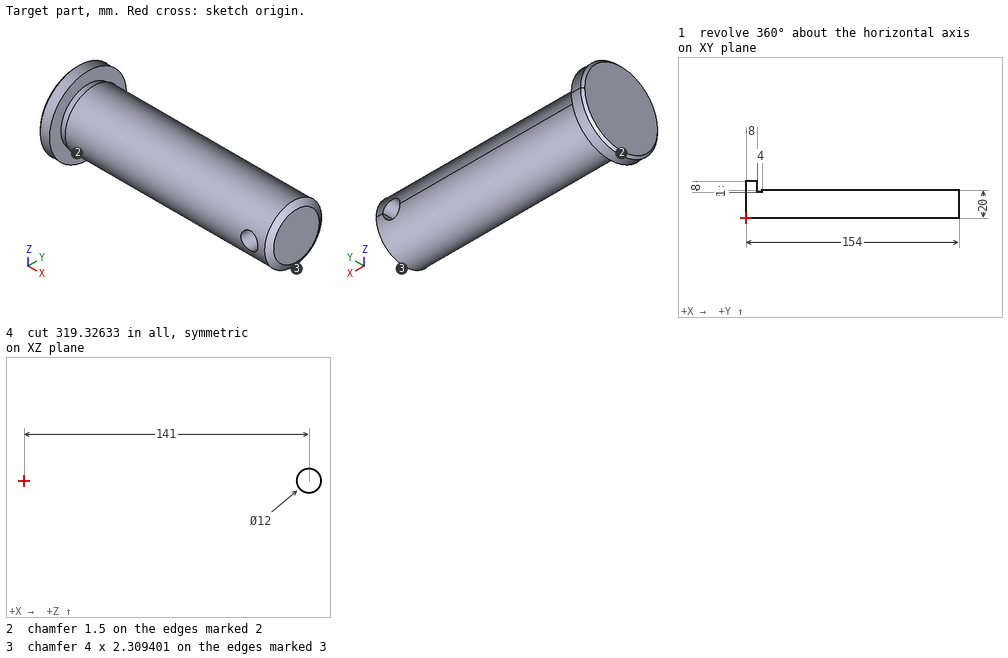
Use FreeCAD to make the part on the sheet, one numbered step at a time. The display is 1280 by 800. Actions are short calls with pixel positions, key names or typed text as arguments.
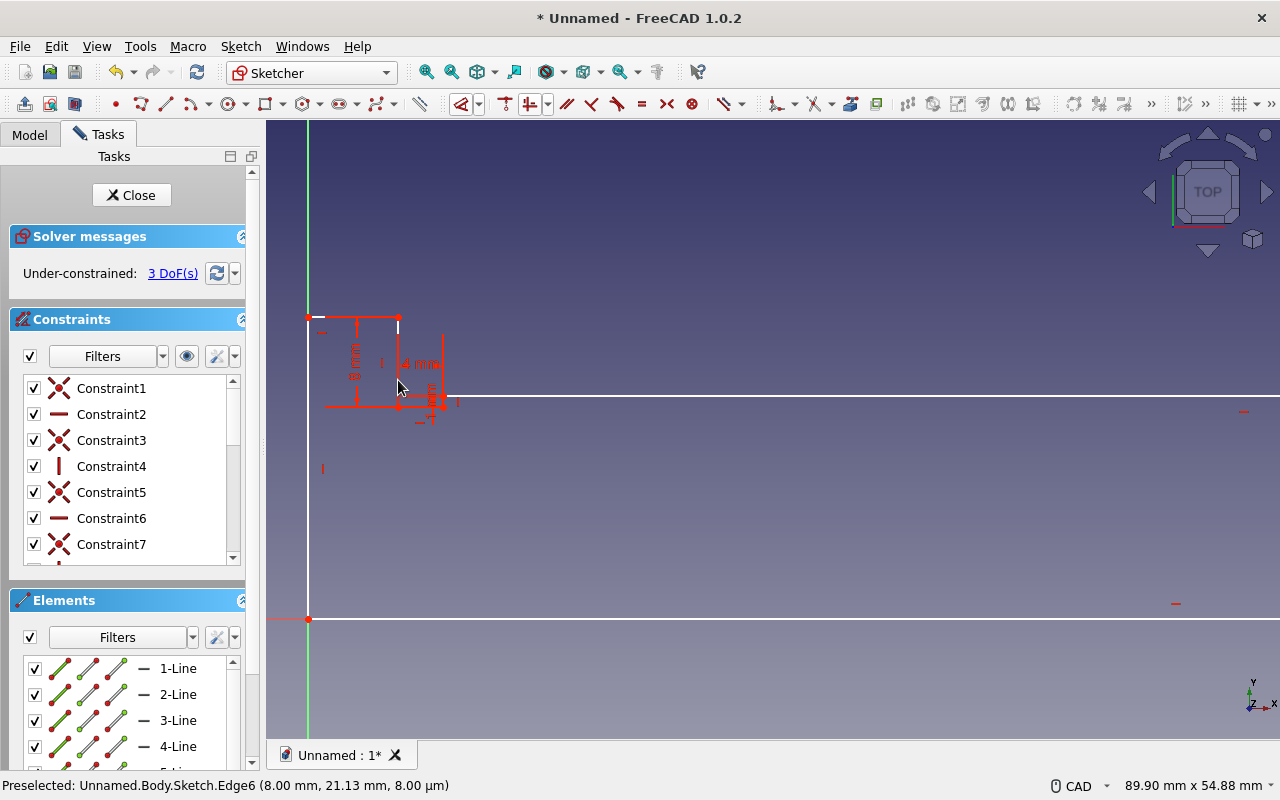
click(371, 317)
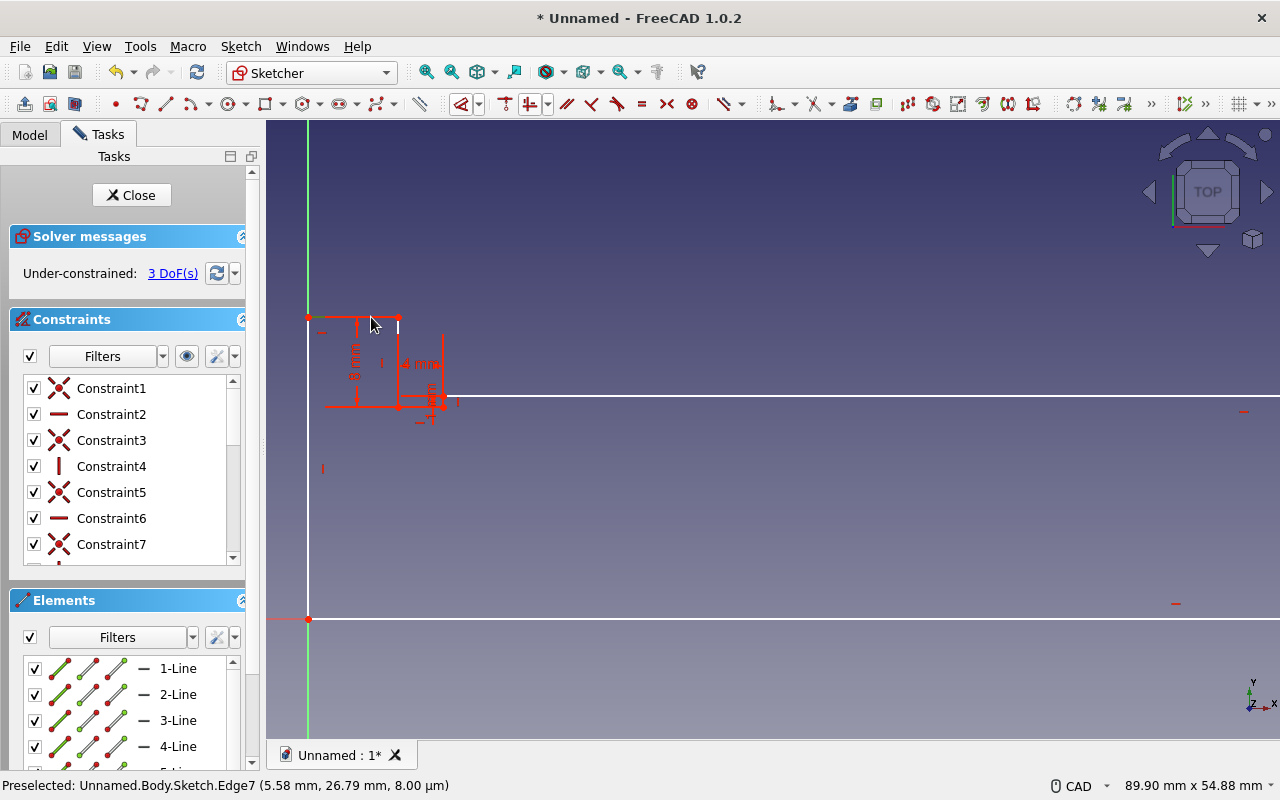
click(478, 104)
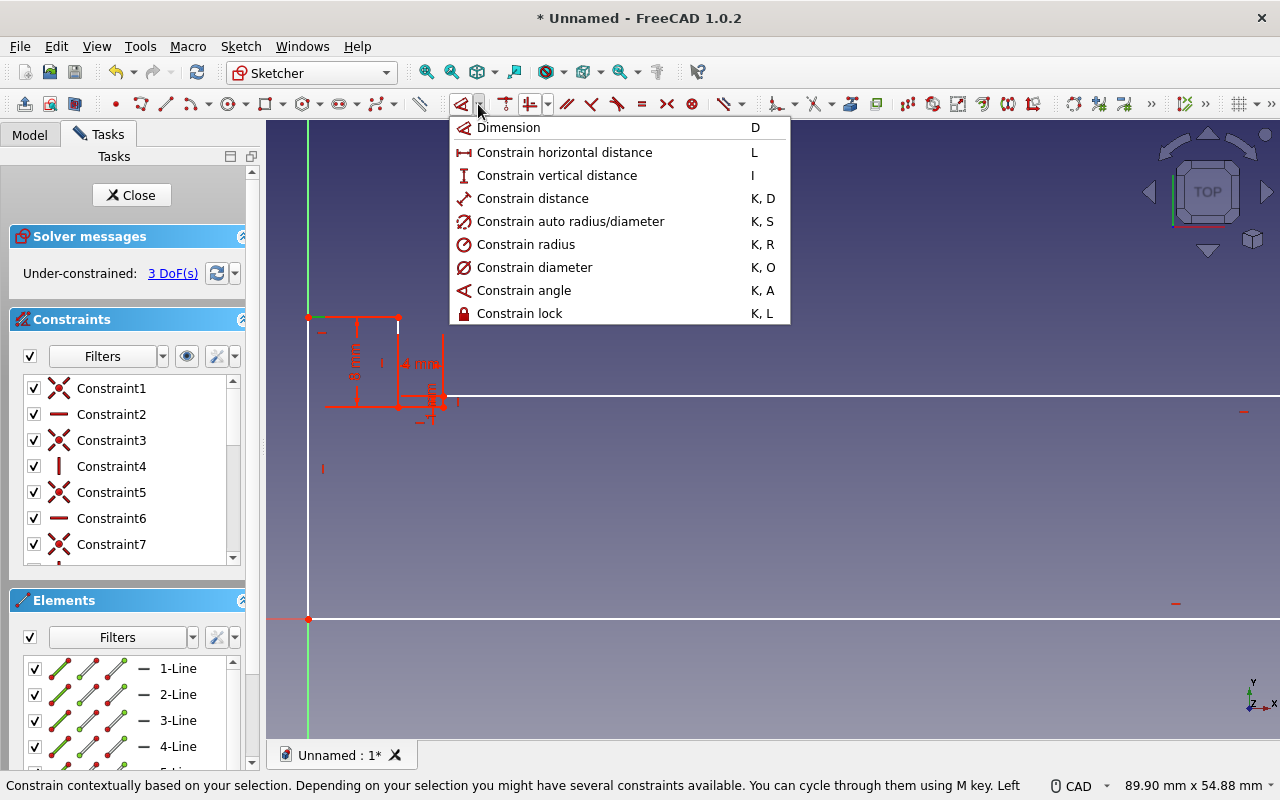
click(620, 152)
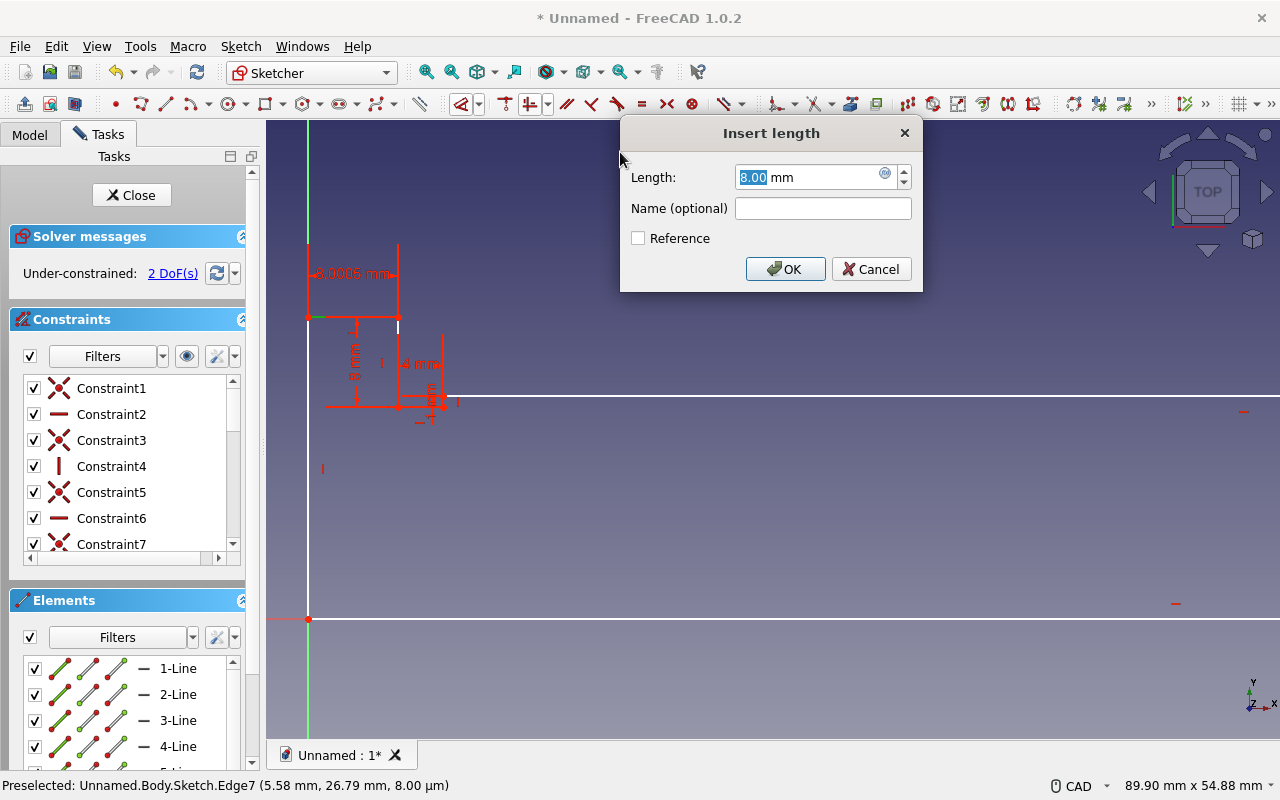
text(8)
key(Return)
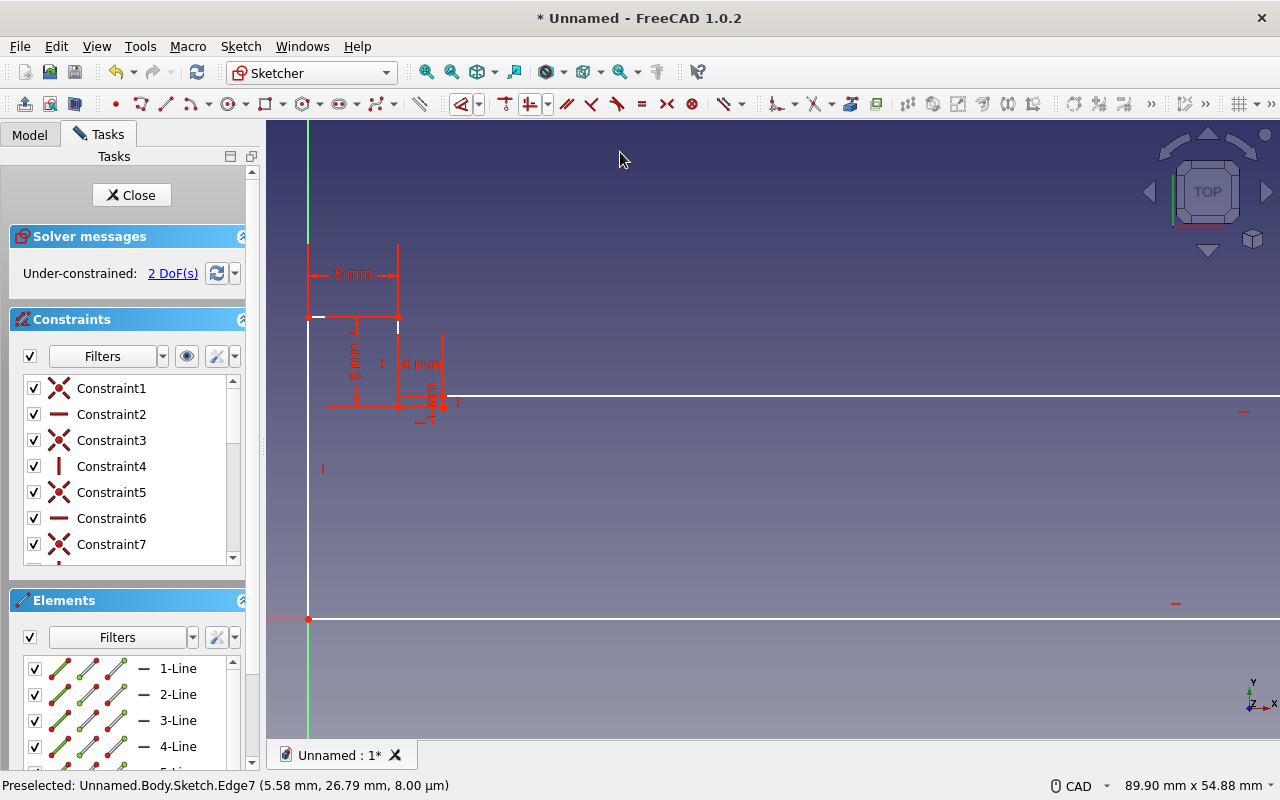
scroll(430, 408, down, 5)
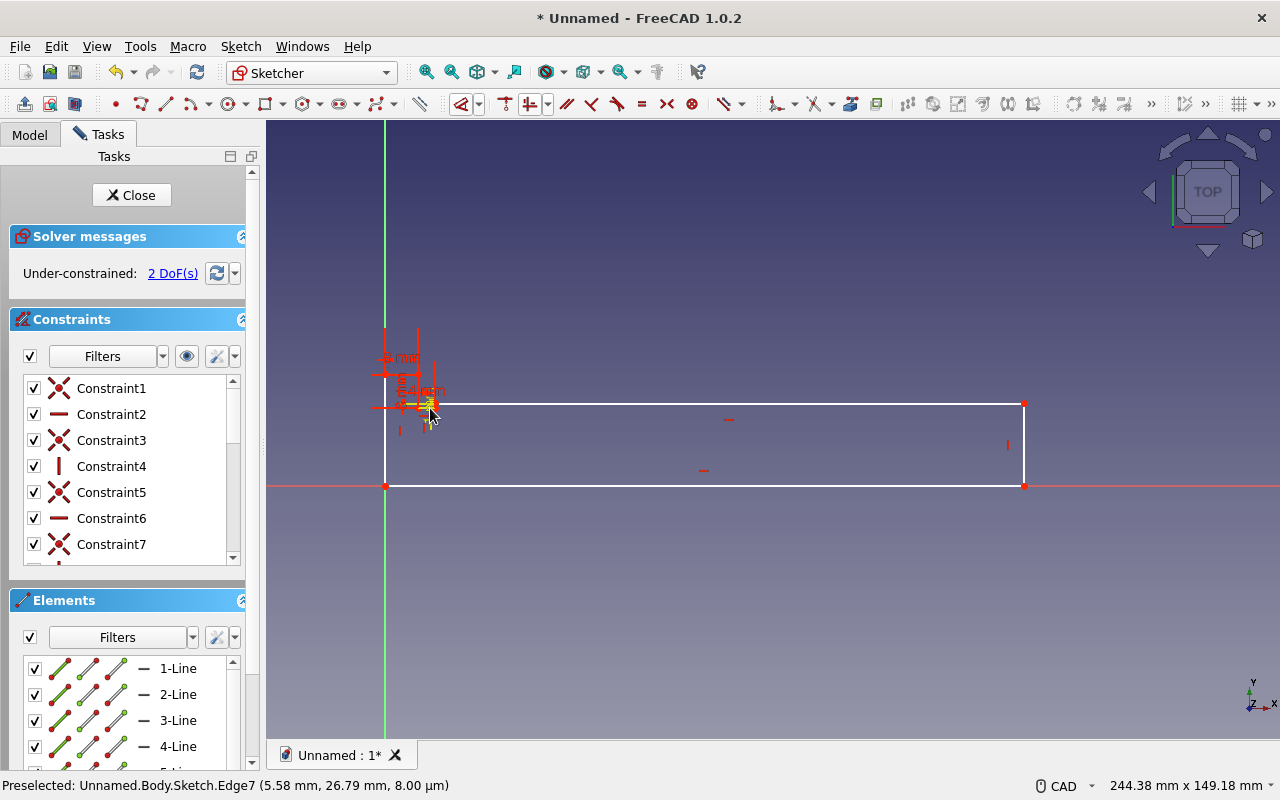
click(1024, 461)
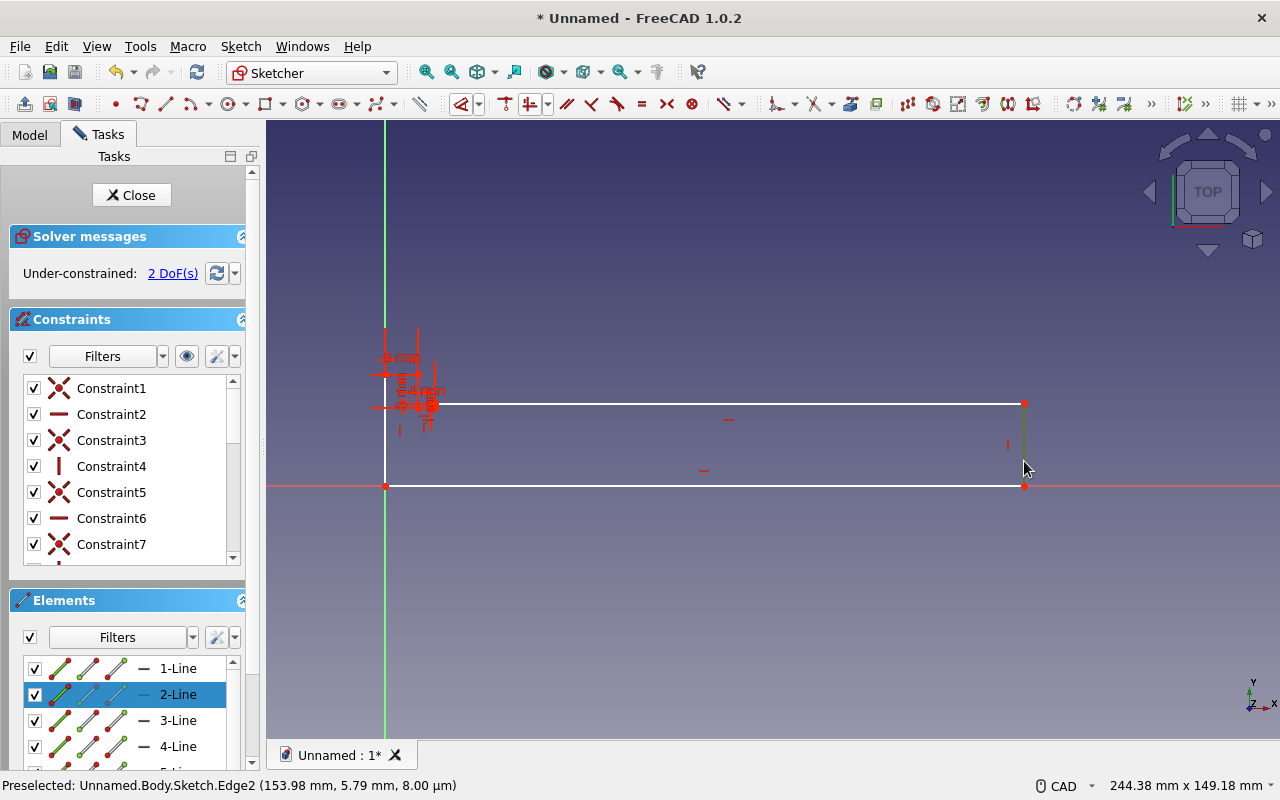
click(478, 104)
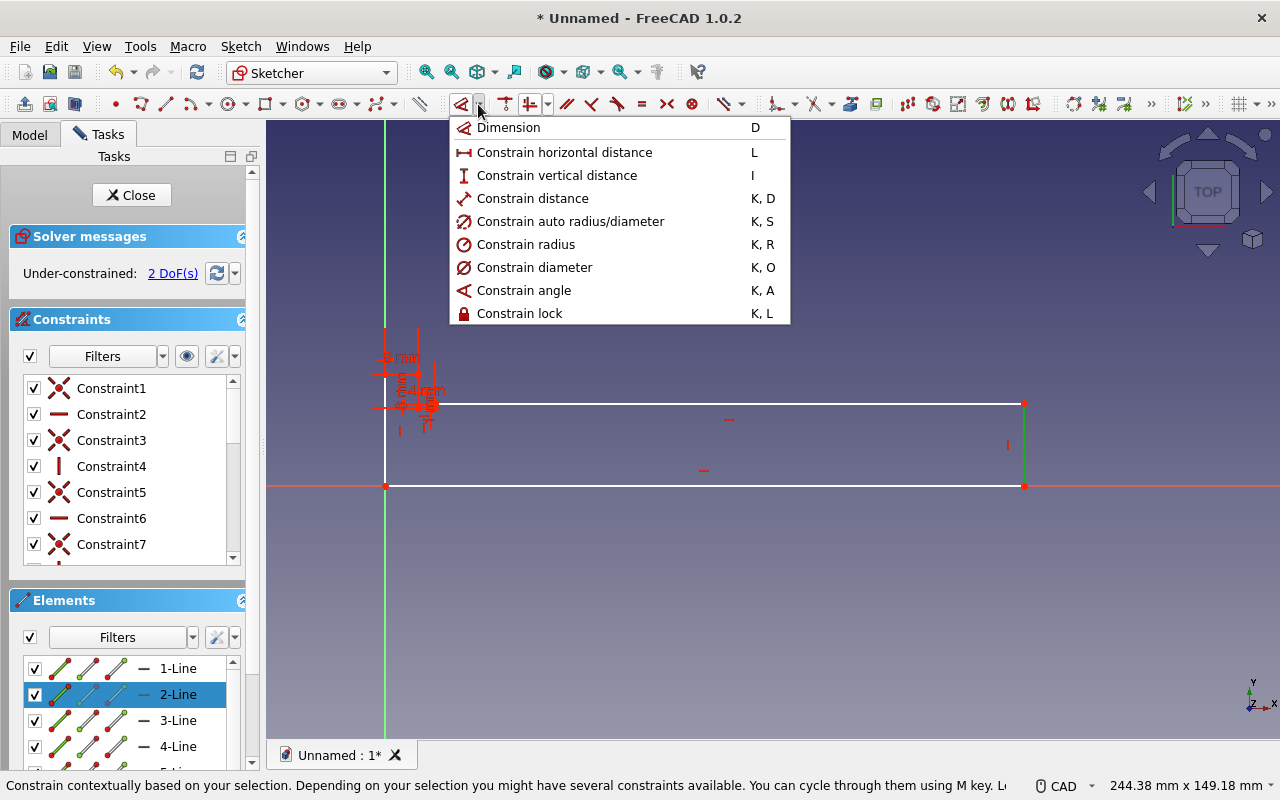
click(620, 176)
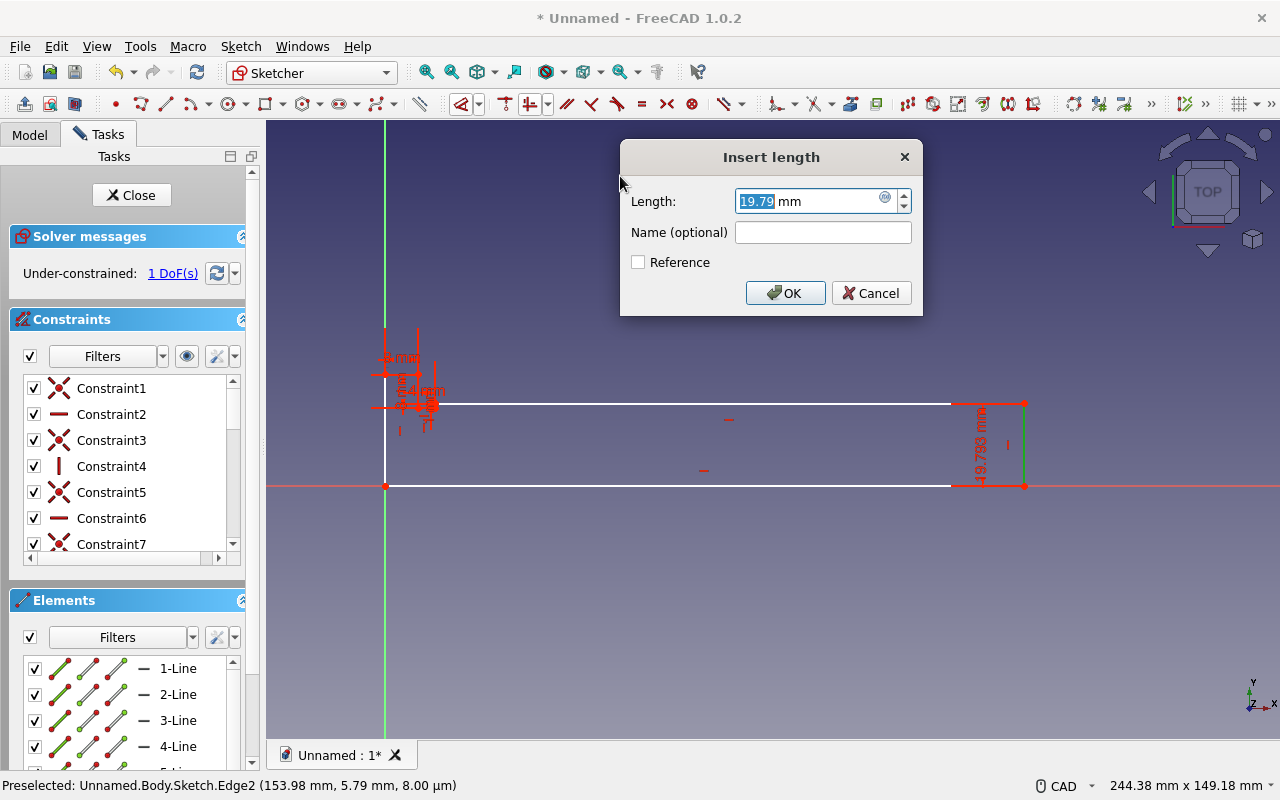
text(20)
key(Return)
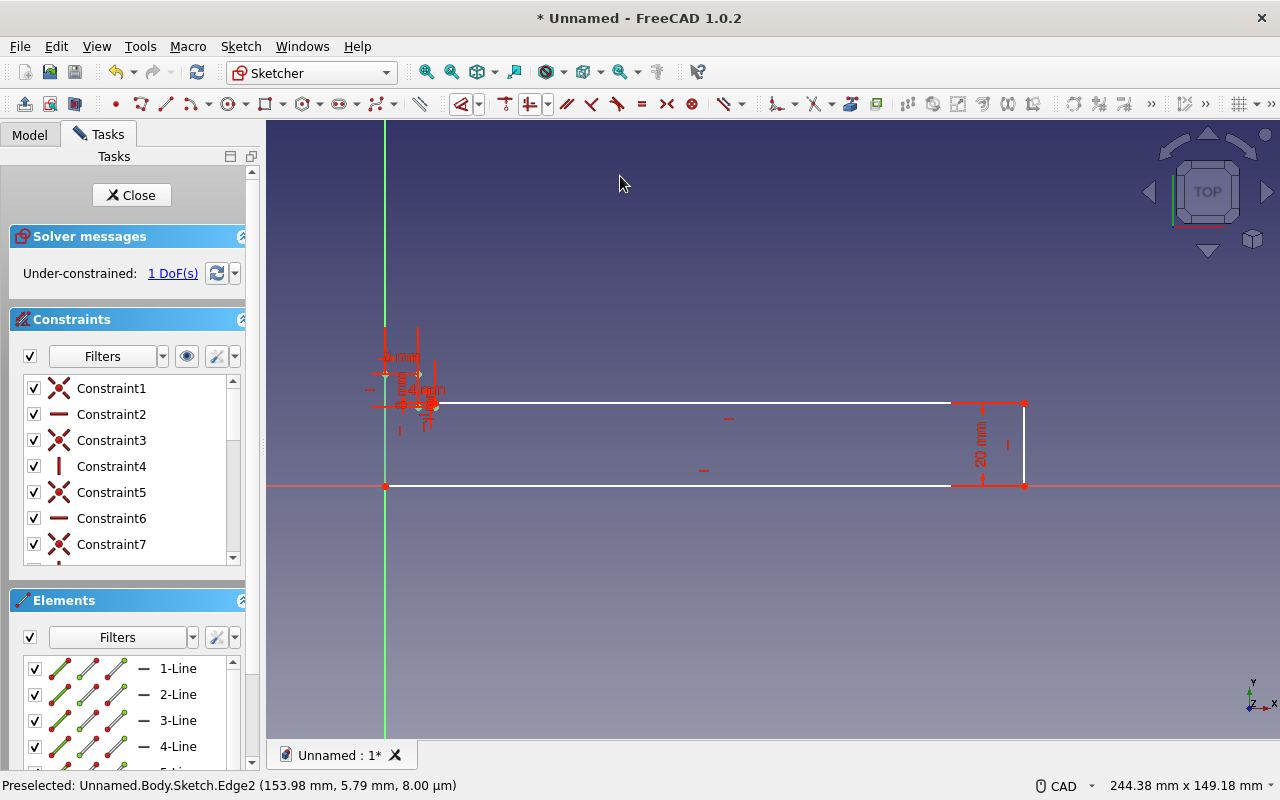
click(577, 486)